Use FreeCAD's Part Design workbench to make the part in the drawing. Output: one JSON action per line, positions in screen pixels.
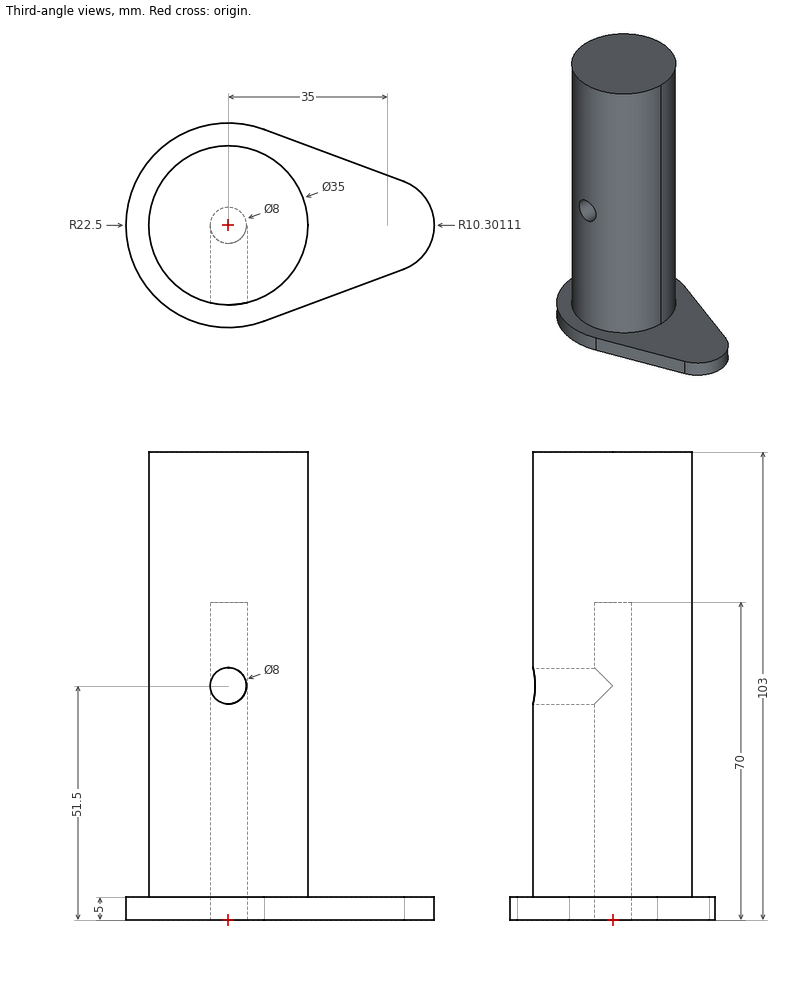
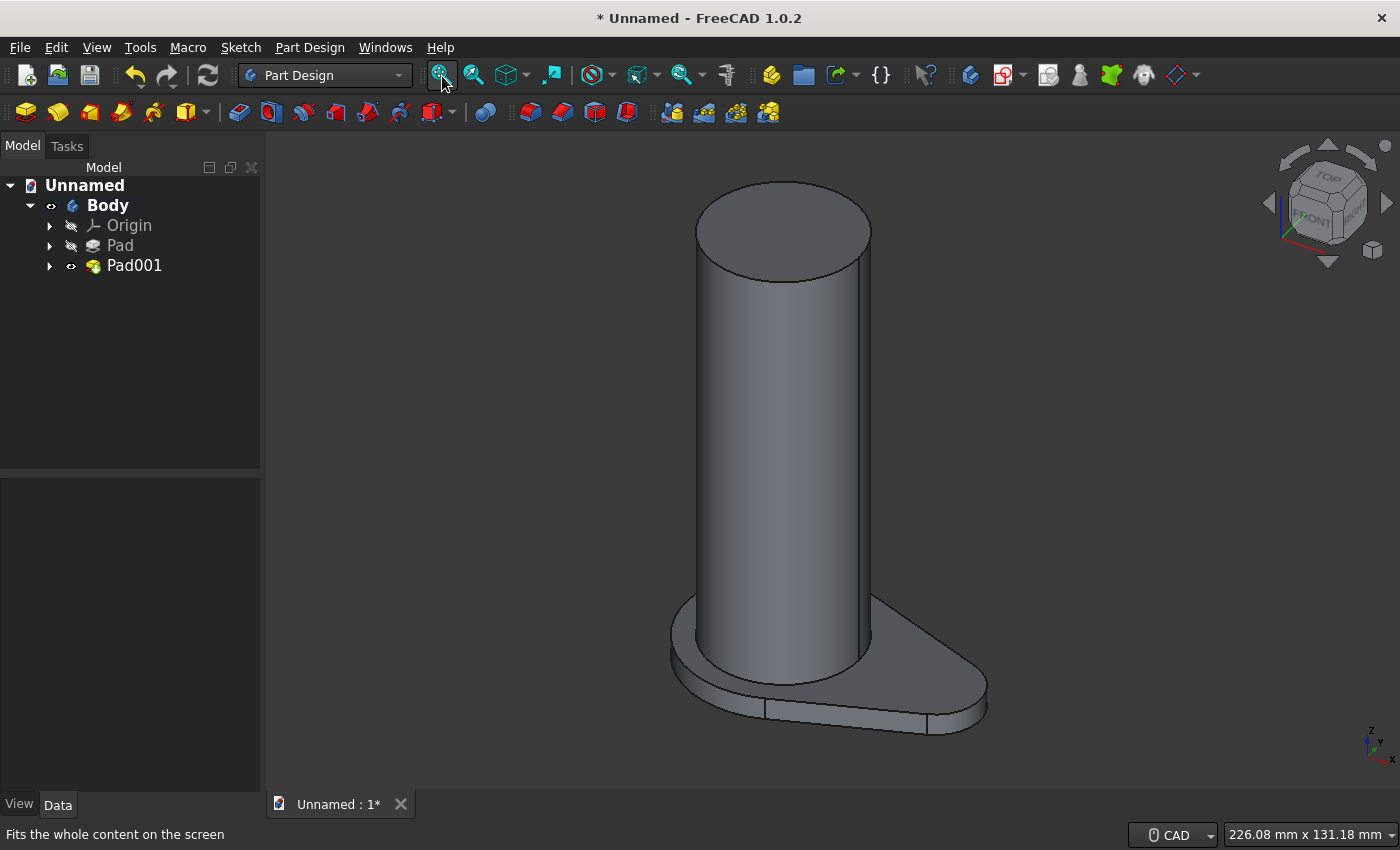
{"action": "left_click", "coordinate": [1004, 76]}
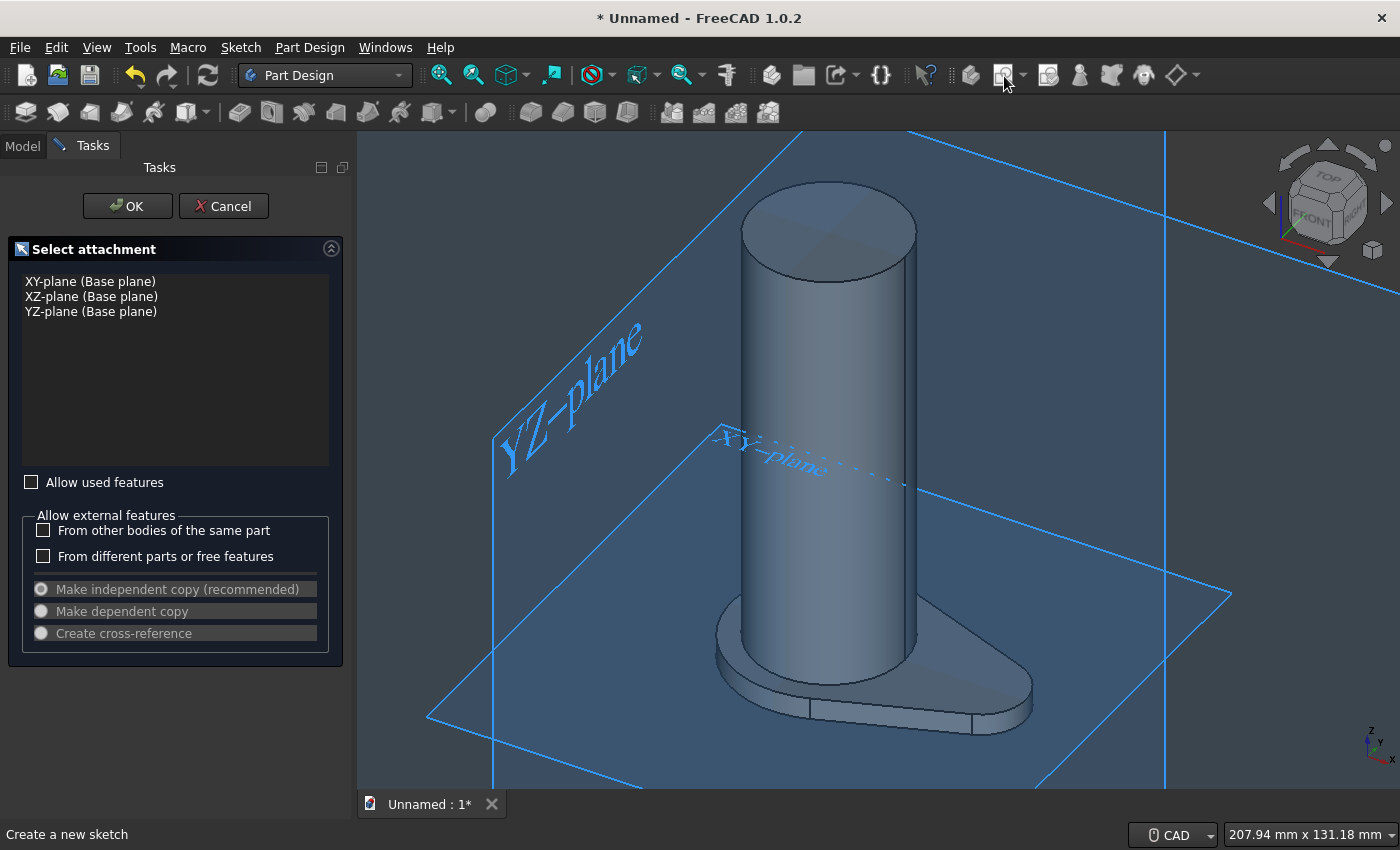
{"action": "left_click", "coordinate": [82, 282]}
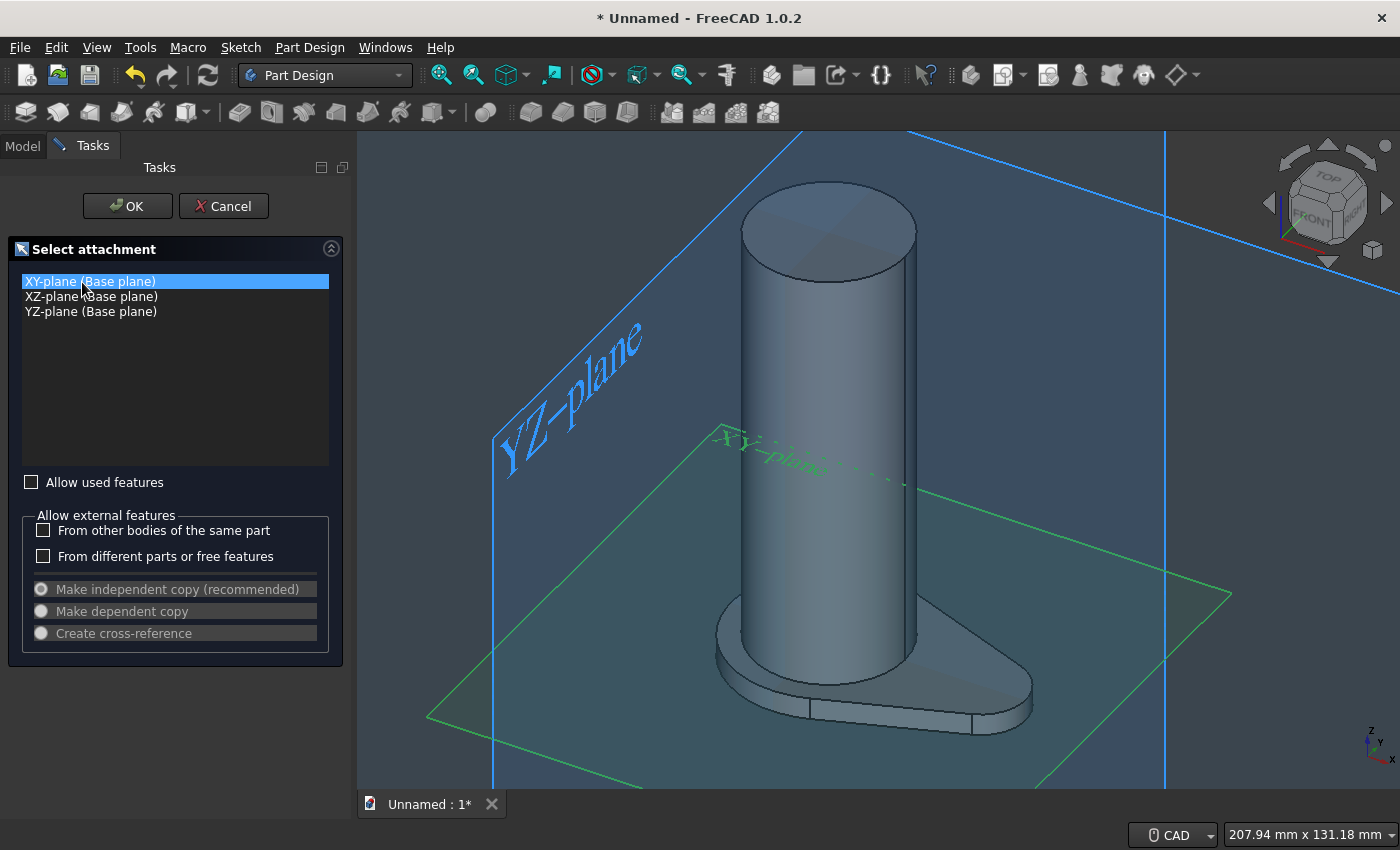
{"action": "left_click", "coordinate": [128, 206]}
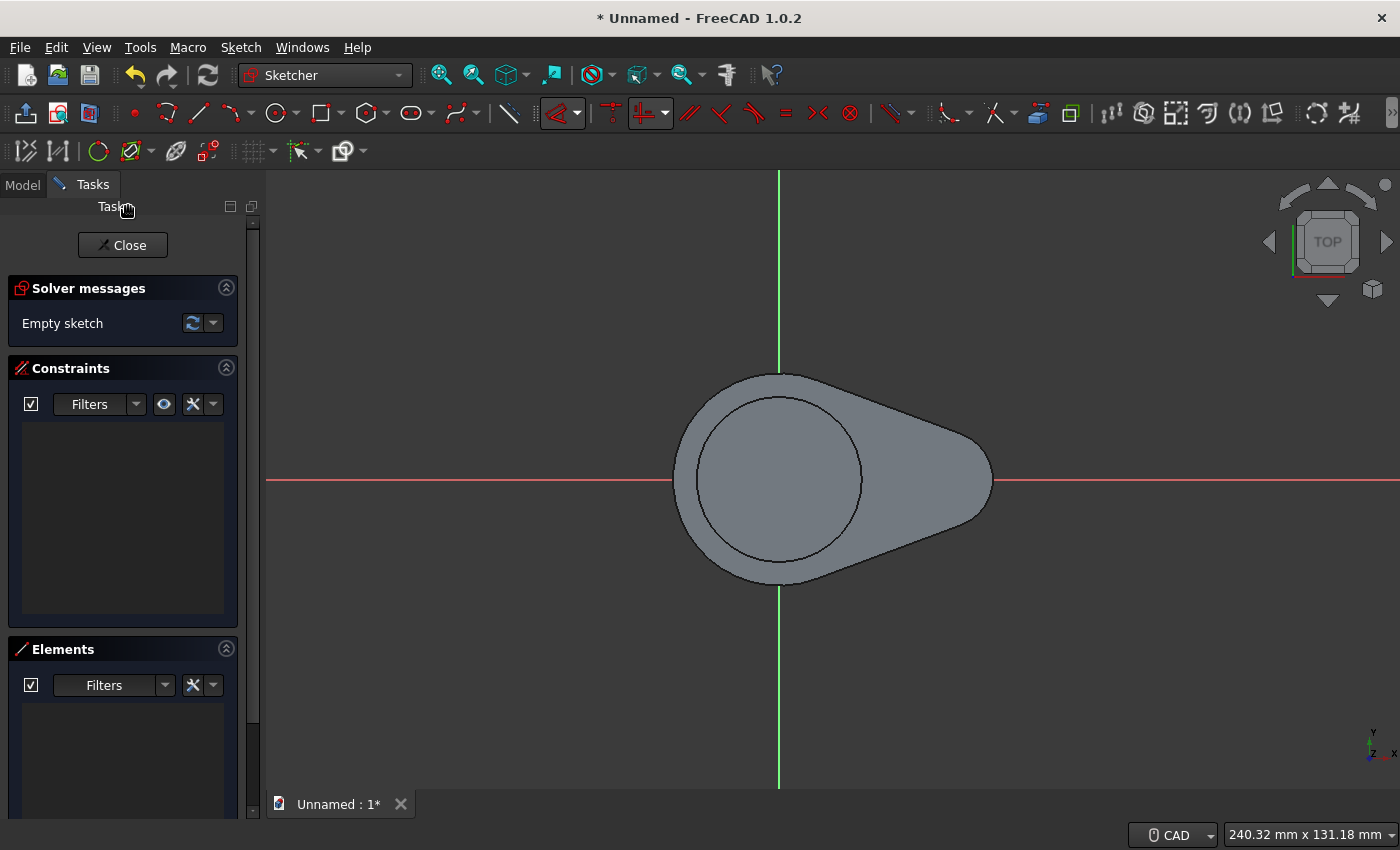
{"action": "left_click", "coordinate": [90, 114]}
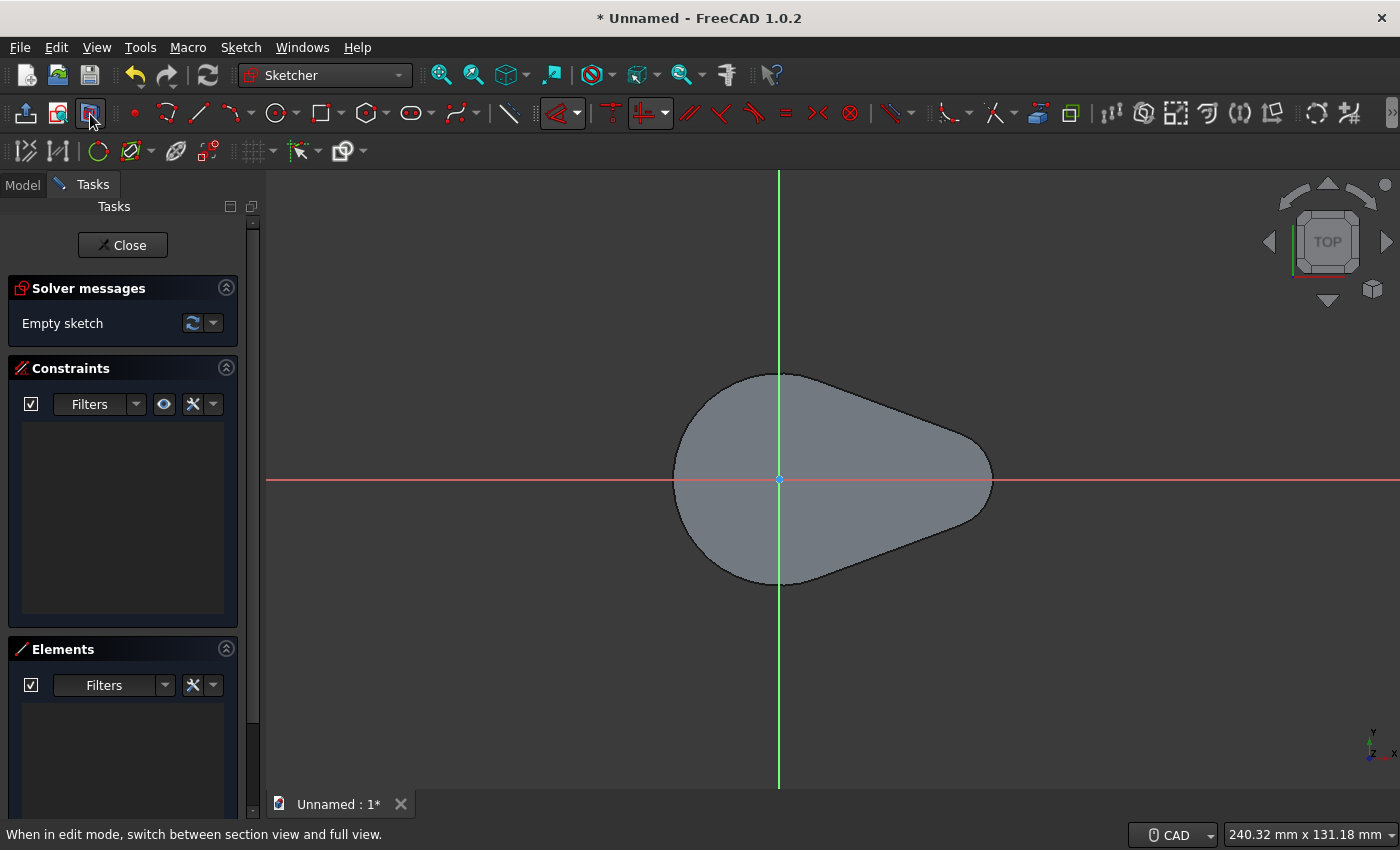
{"action": "scroll", "coordinate": [781, 480], "scroll_direction": "up", "scroll_amount": 12}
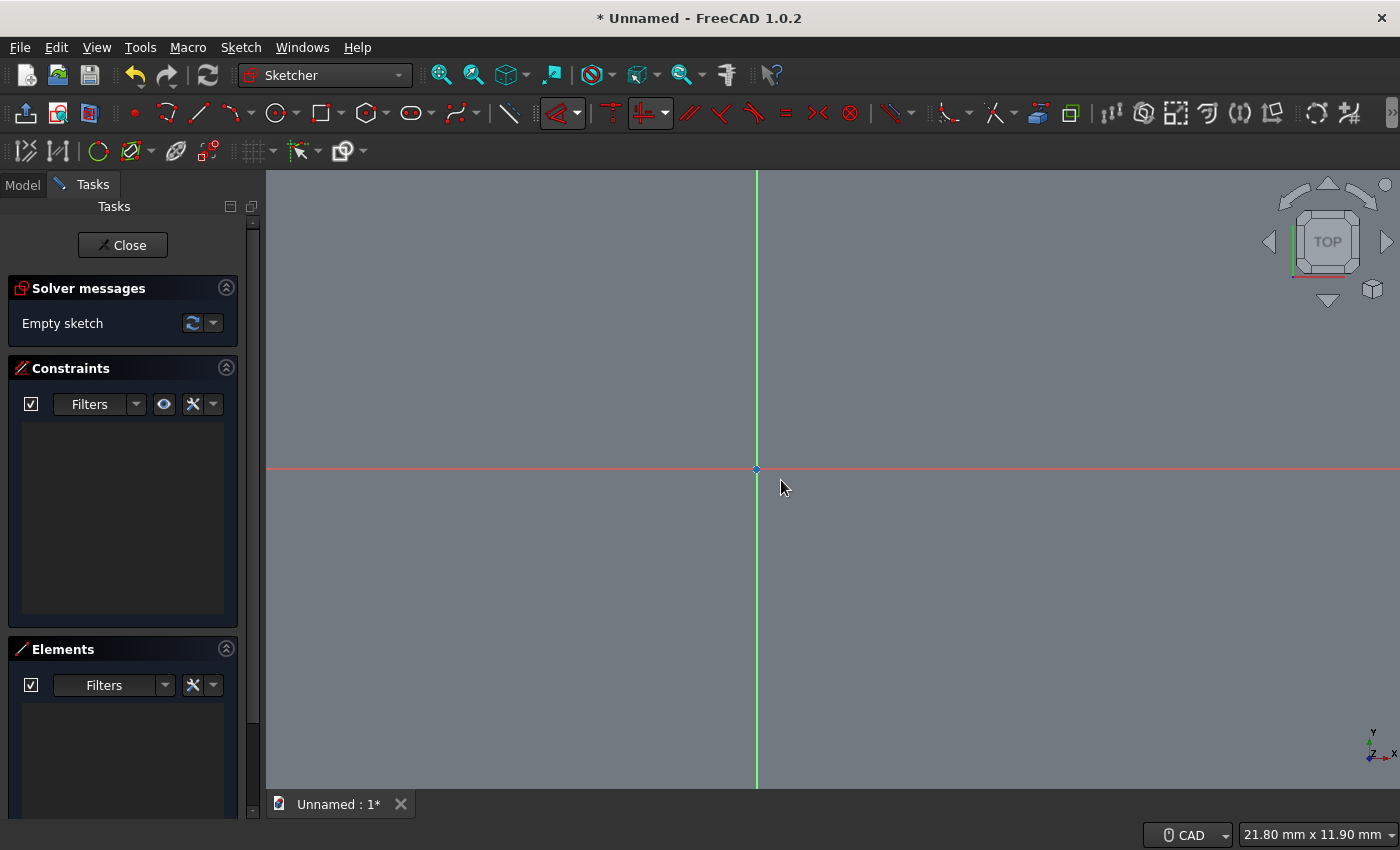
{"action": "left_click", "coordinate": [276, 114]}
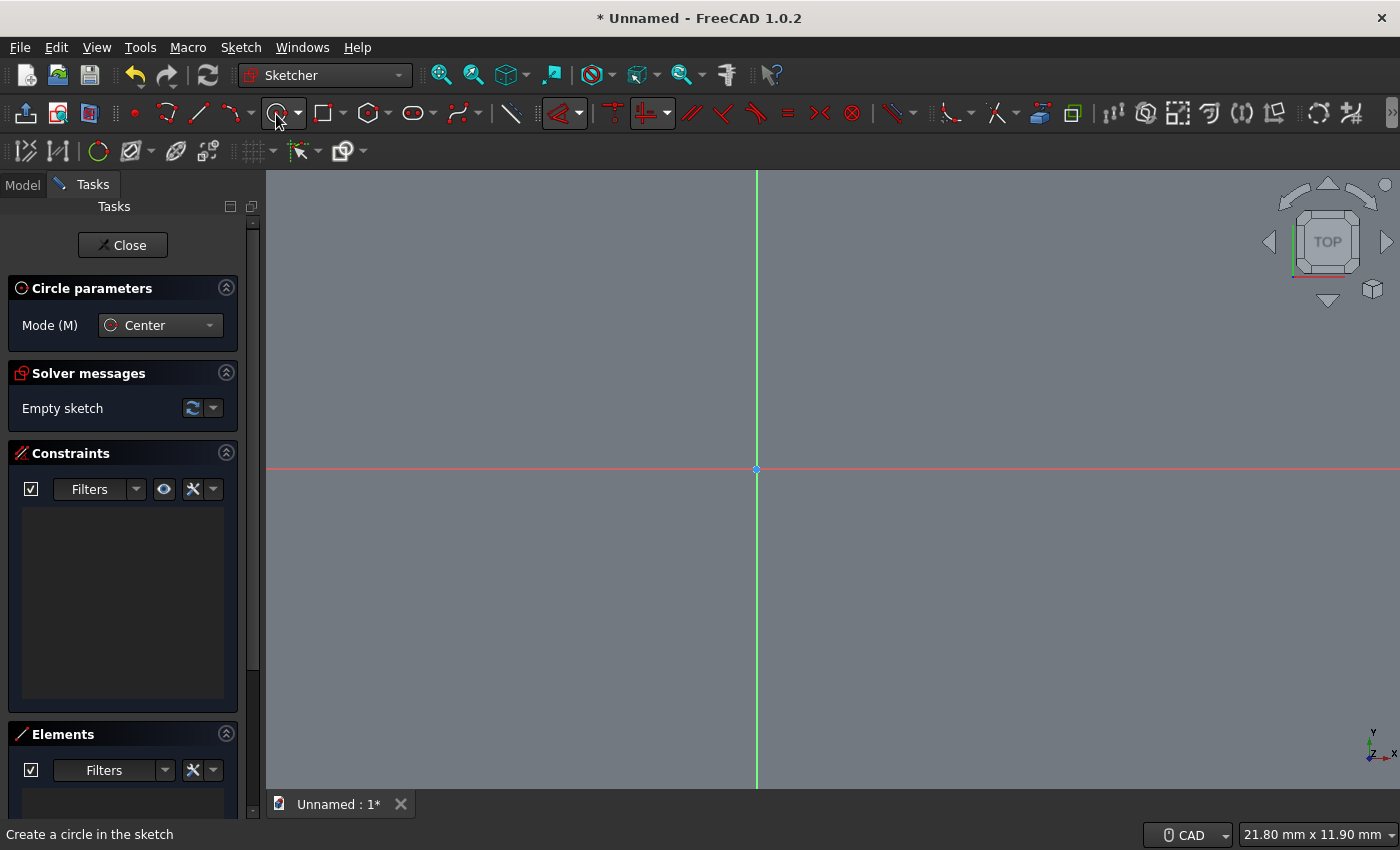
{"action": "left_click", "coordinate": [757, 469]}
{"action": "left_click", "coordinate": [904, 322]}
{"action": "key", "text": "Escape"}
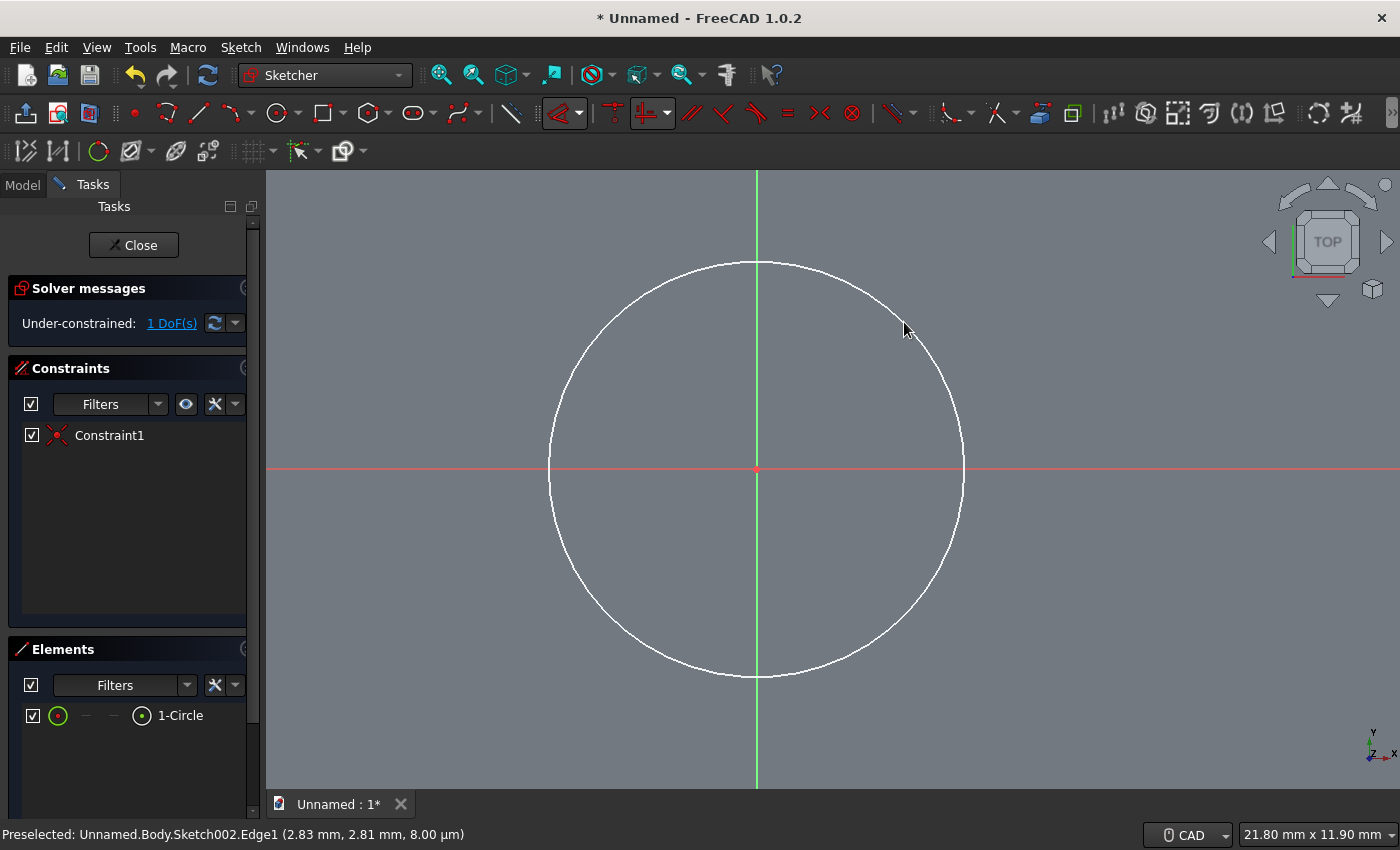
{"action": "left_click", "coordinate": [903, 322]}